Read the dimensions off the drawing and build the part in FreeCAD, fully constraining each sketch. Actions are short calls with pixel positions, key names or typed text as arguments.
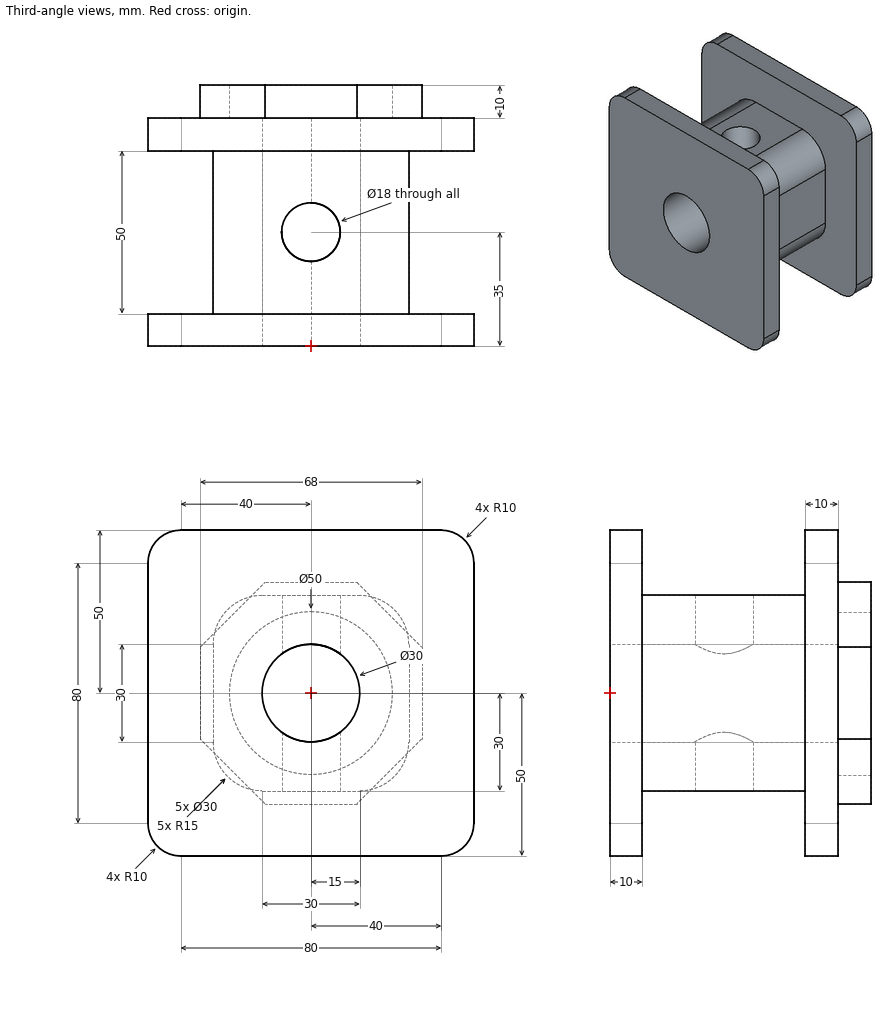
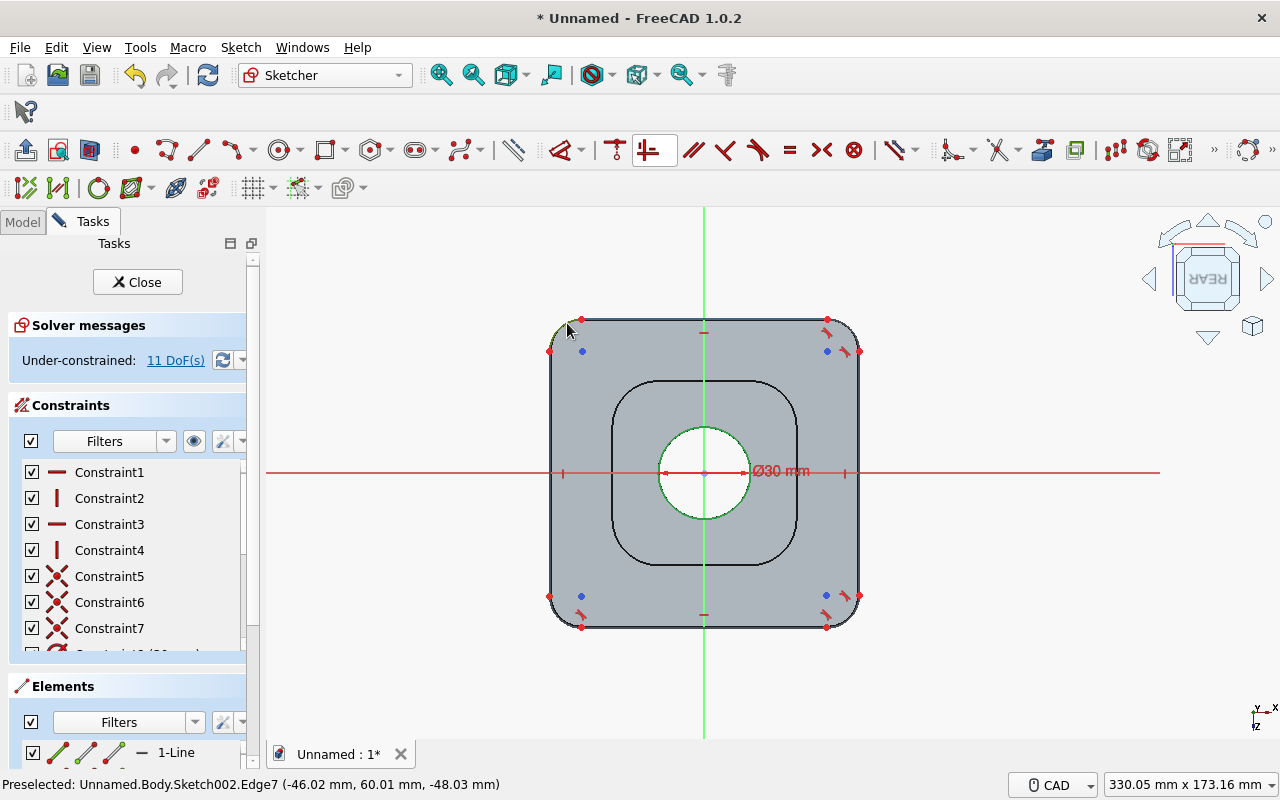
click(758, 150)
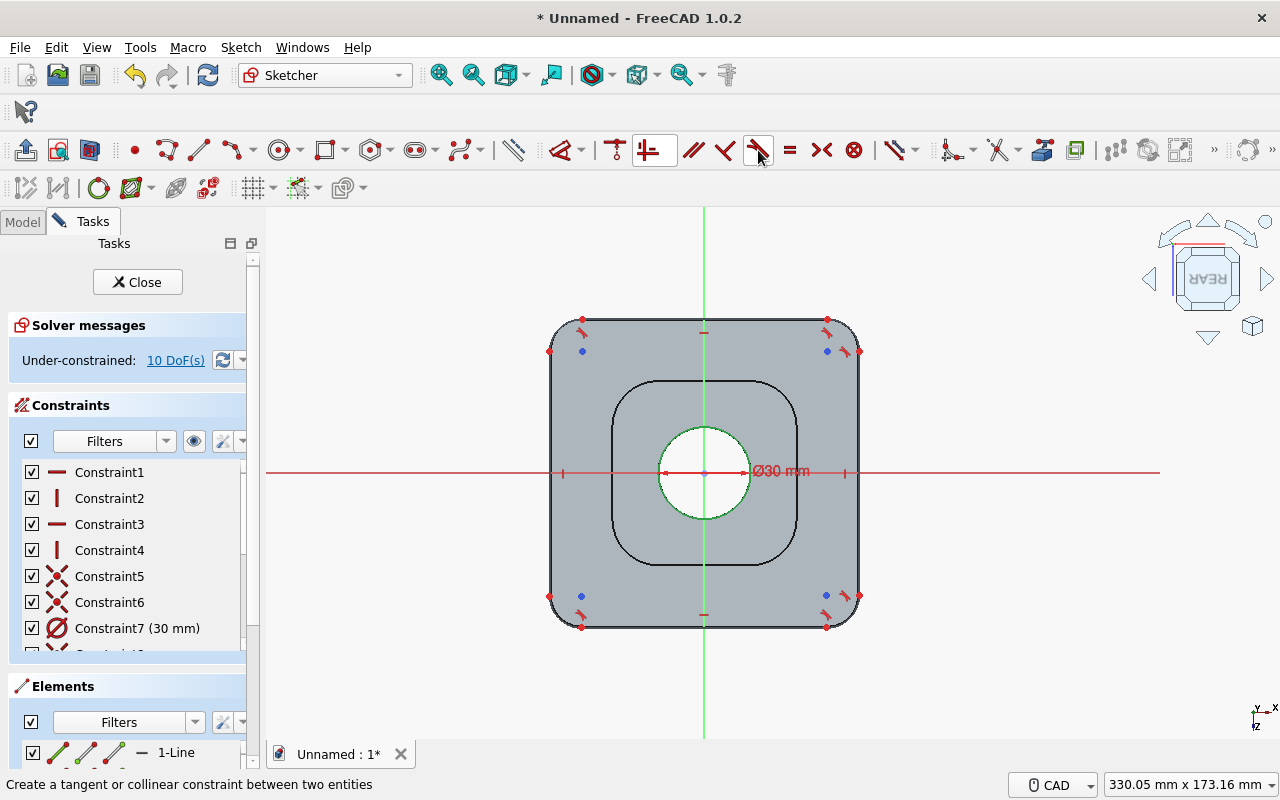
click(550, 425)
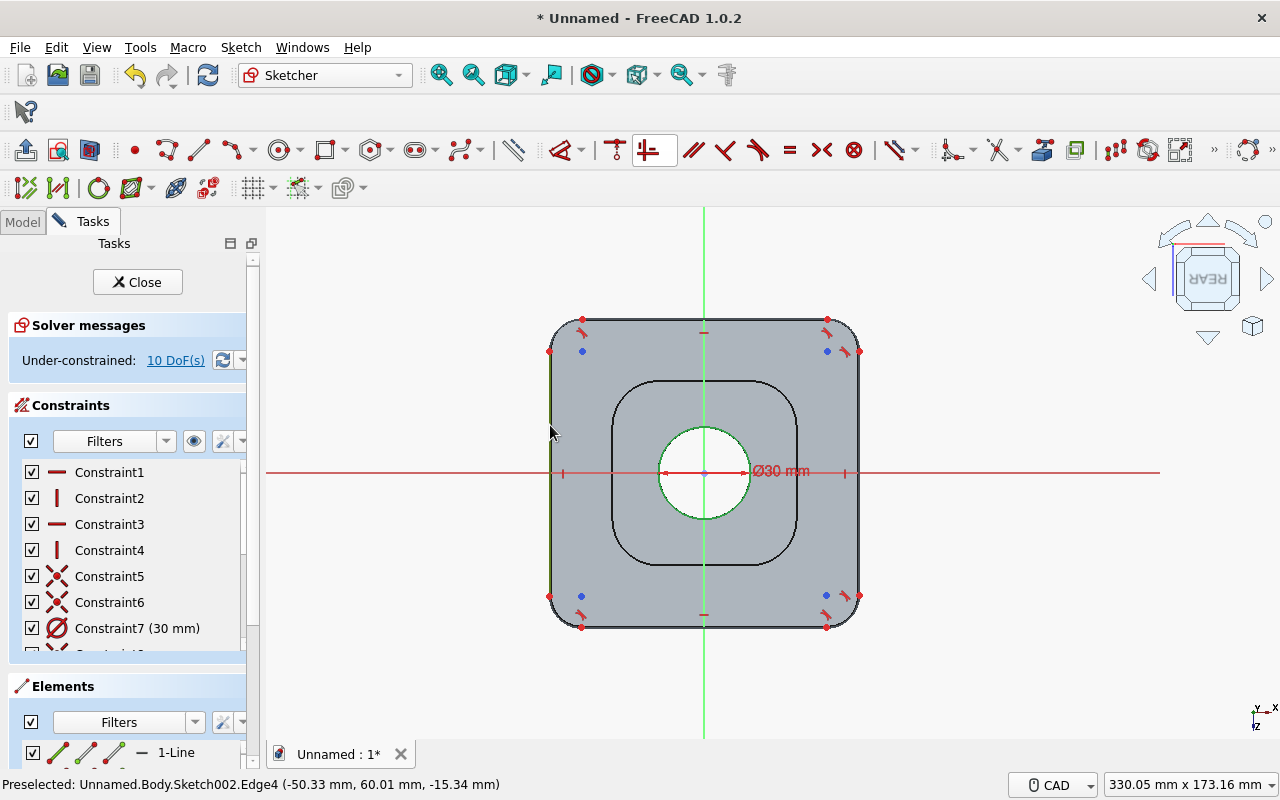
click(568, 323)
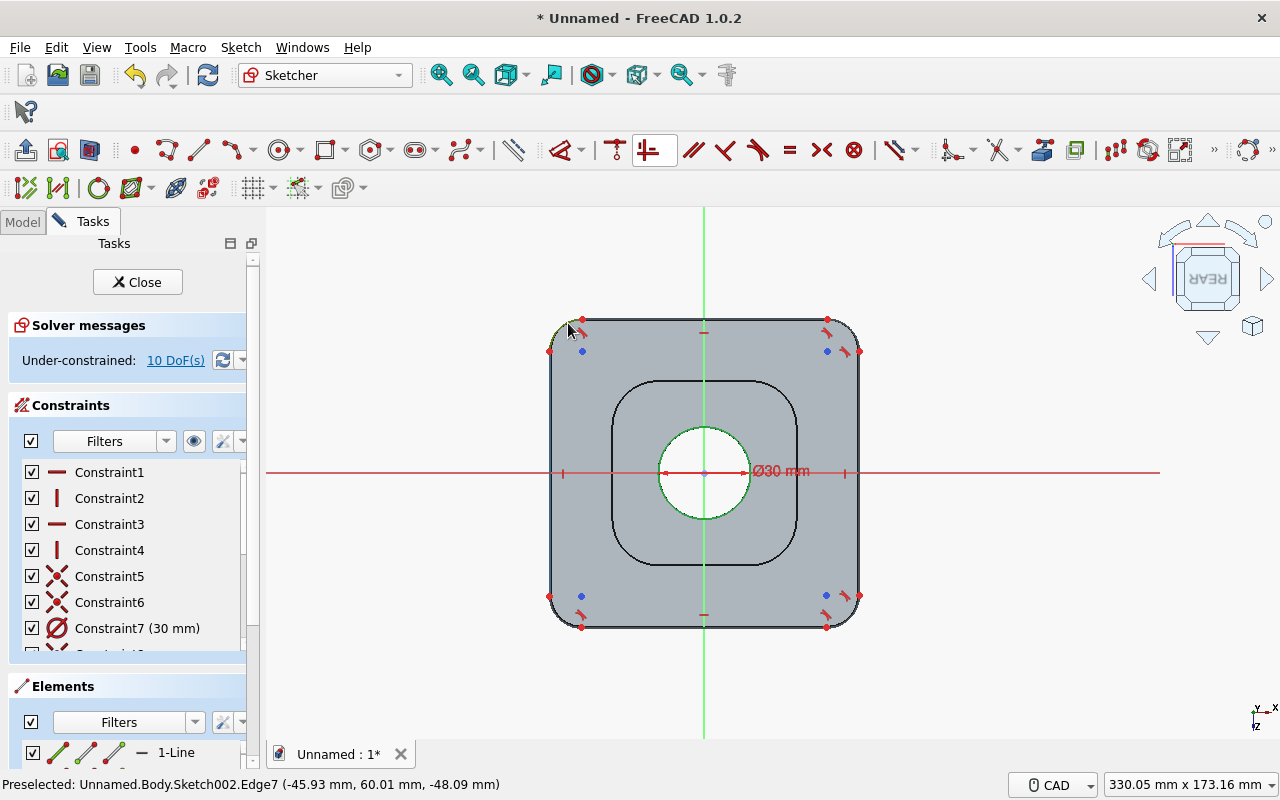
click(758, 150)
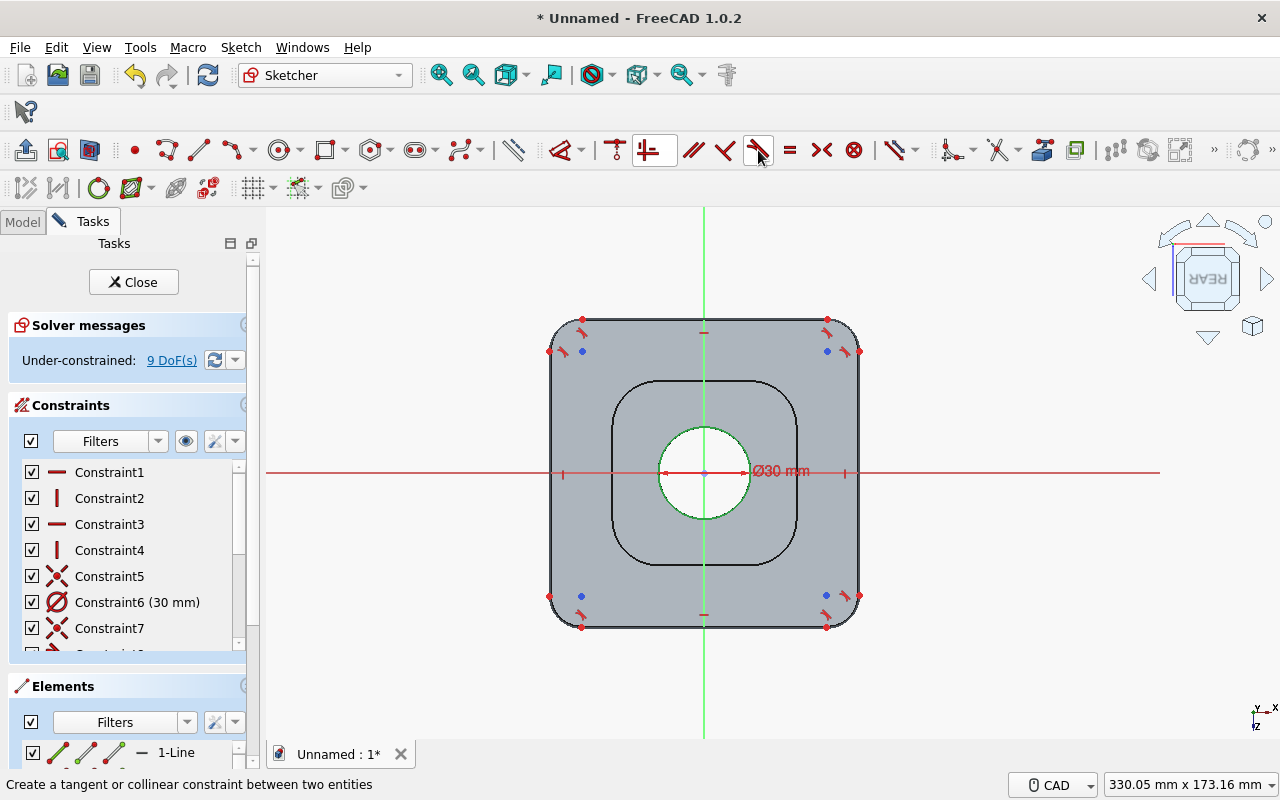
click(550, 425)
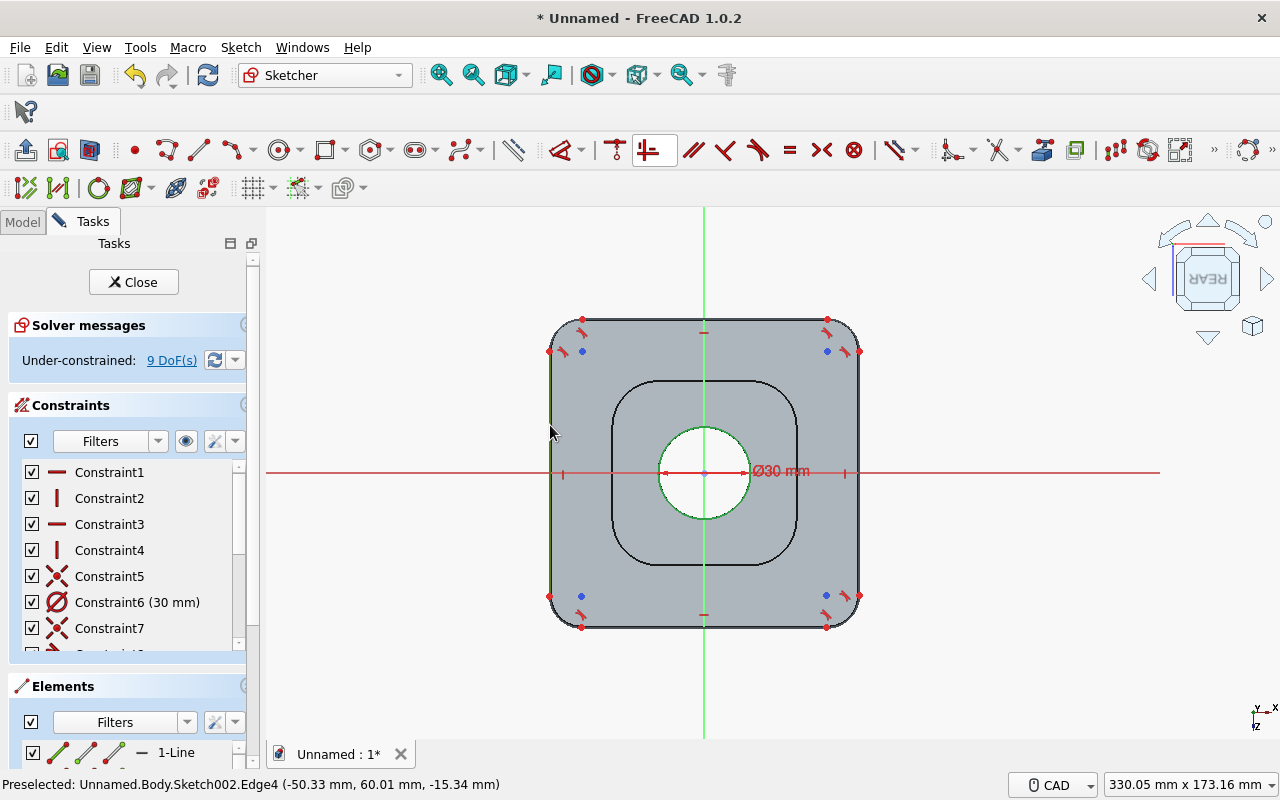
click(554, 611)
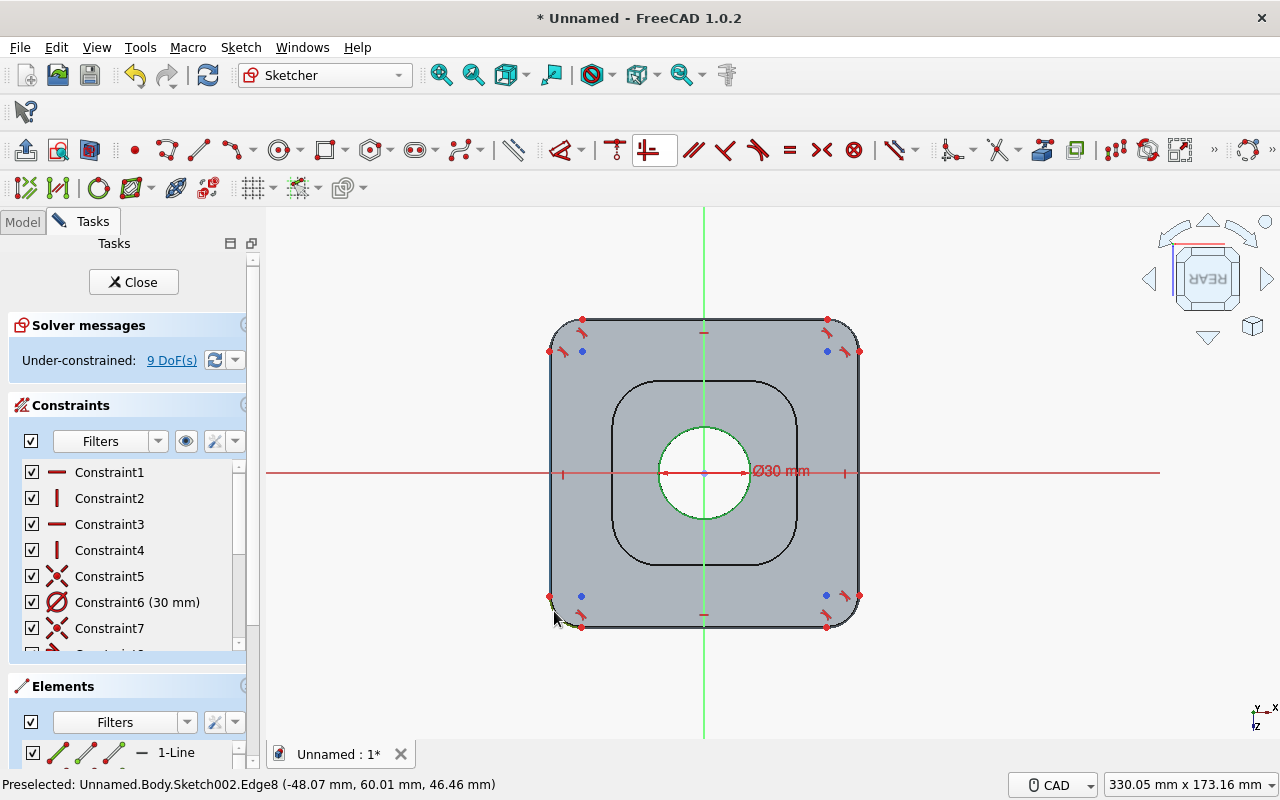
click(758, 150)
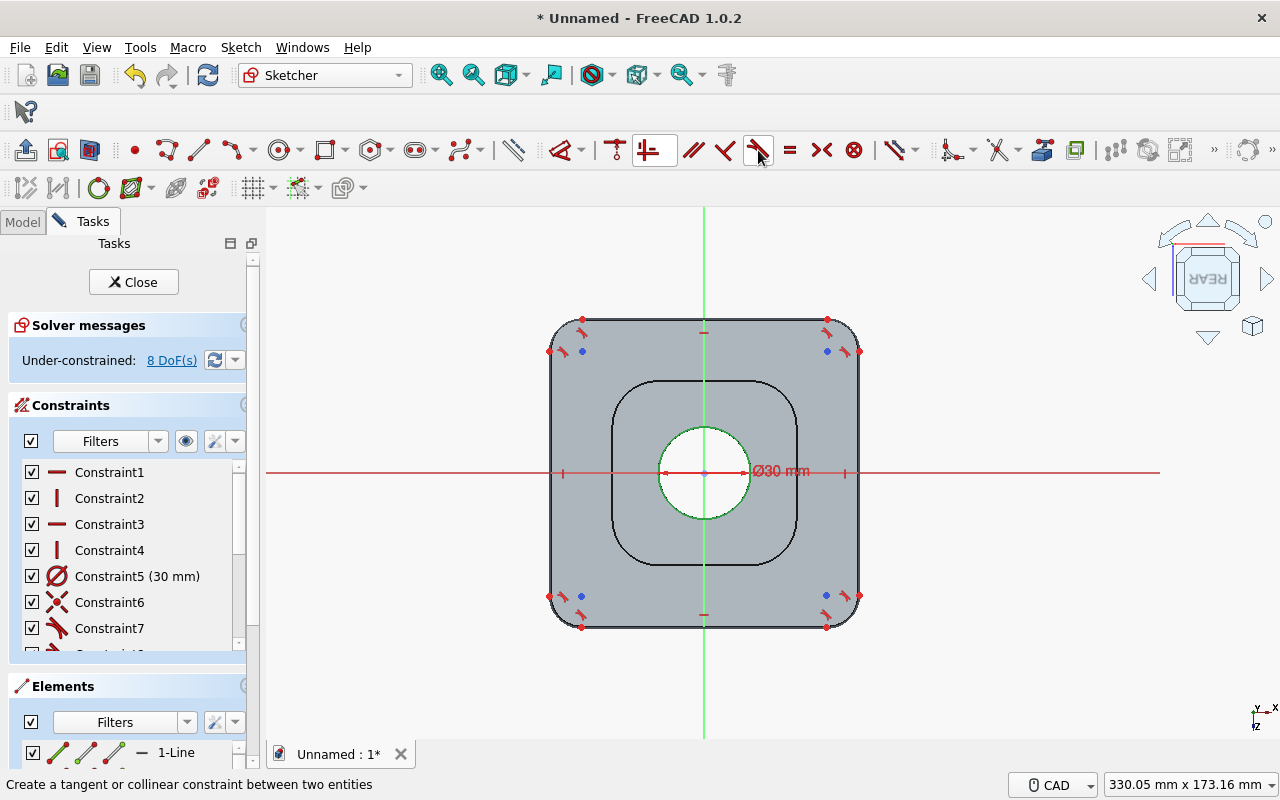
click(841, 624)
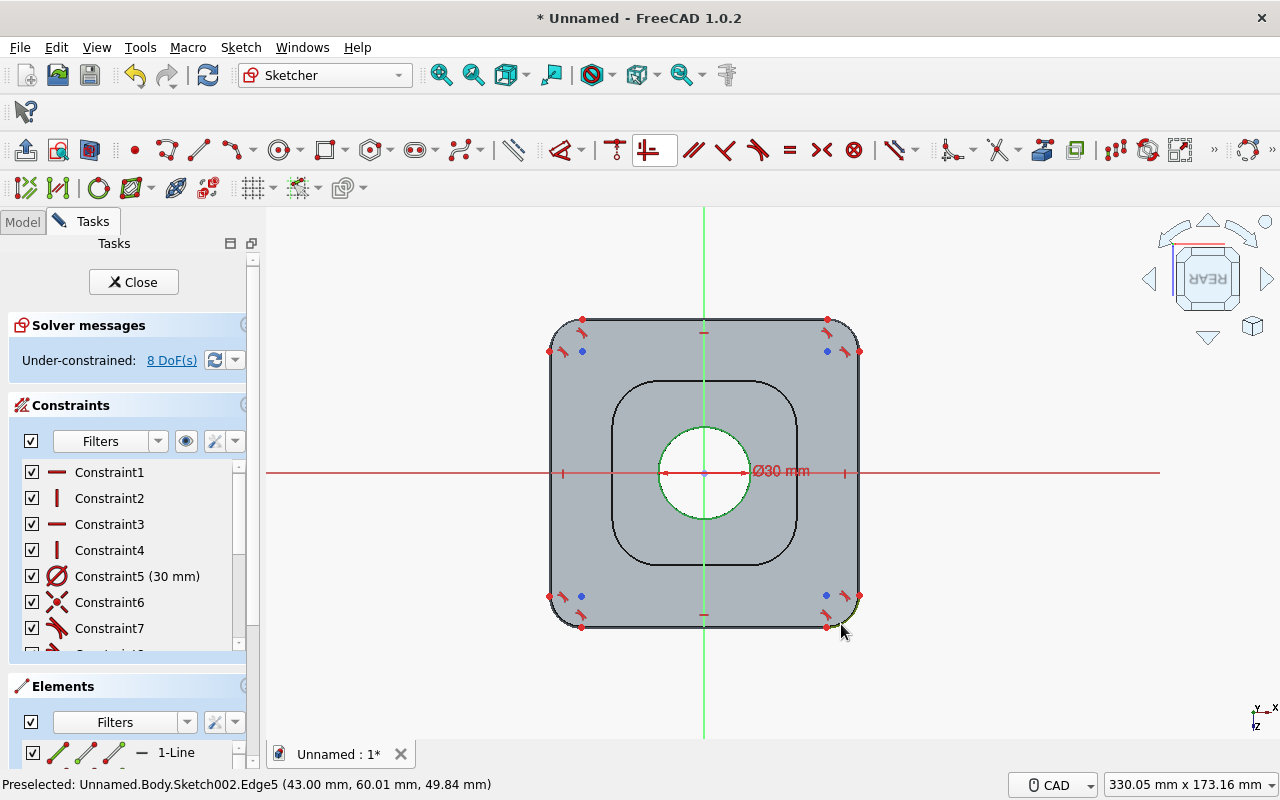
click(856, 337)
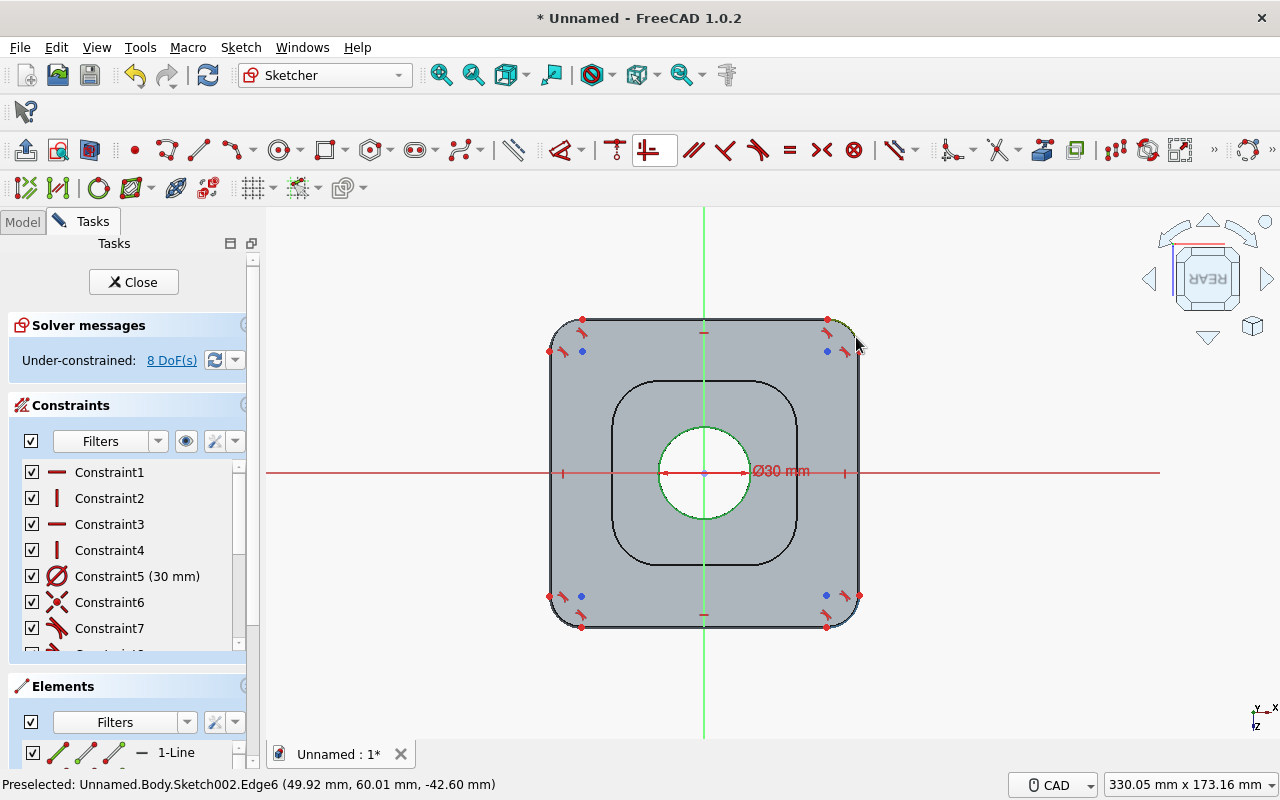
click(568, 323)